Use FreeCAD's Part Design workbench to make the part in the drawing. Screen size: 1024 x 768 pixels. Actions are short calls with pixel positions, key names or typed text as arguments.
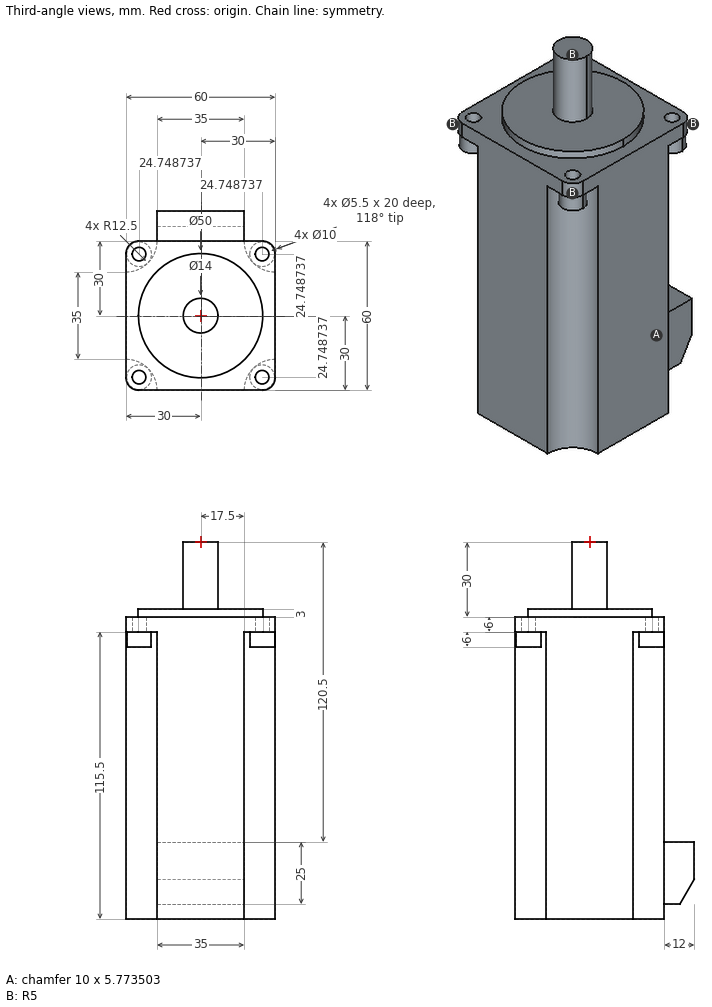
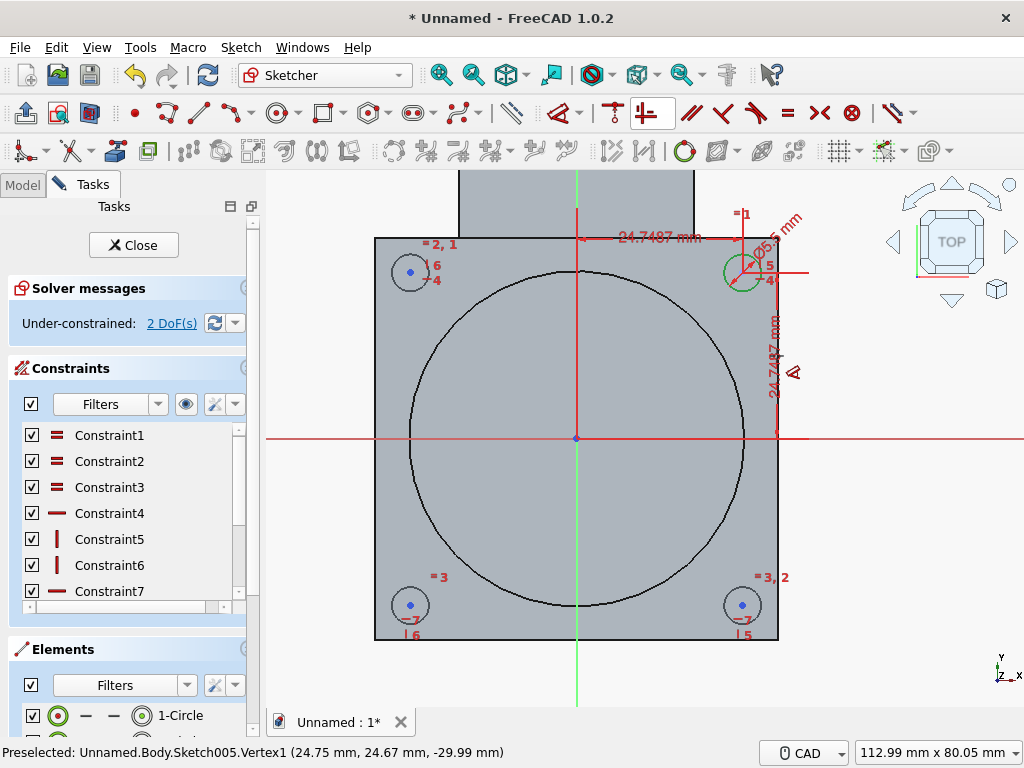
click(410, 273)
click(494, 239)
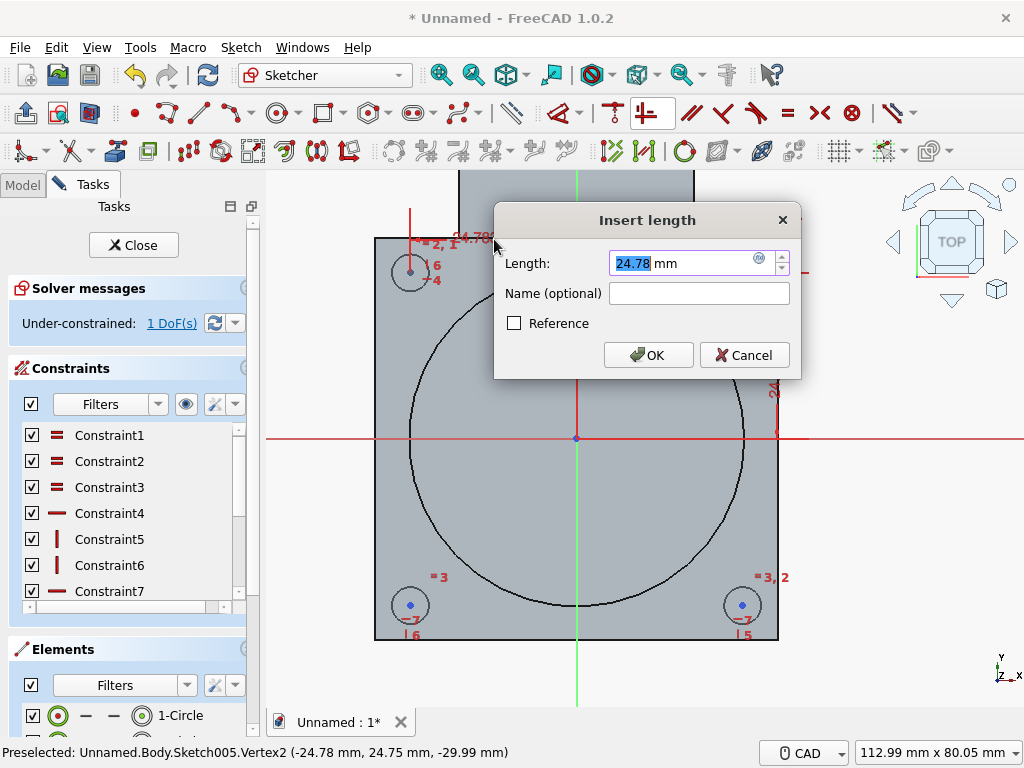
text(24.748737)
key(Return)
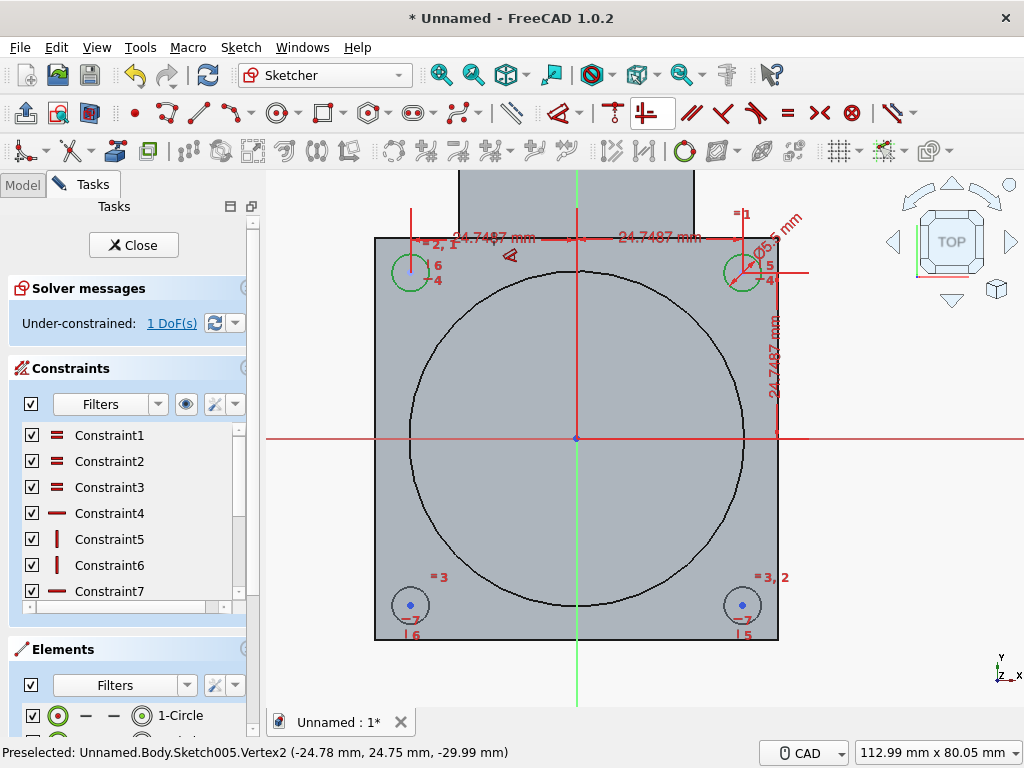
click(743, 606)
click(777, 522)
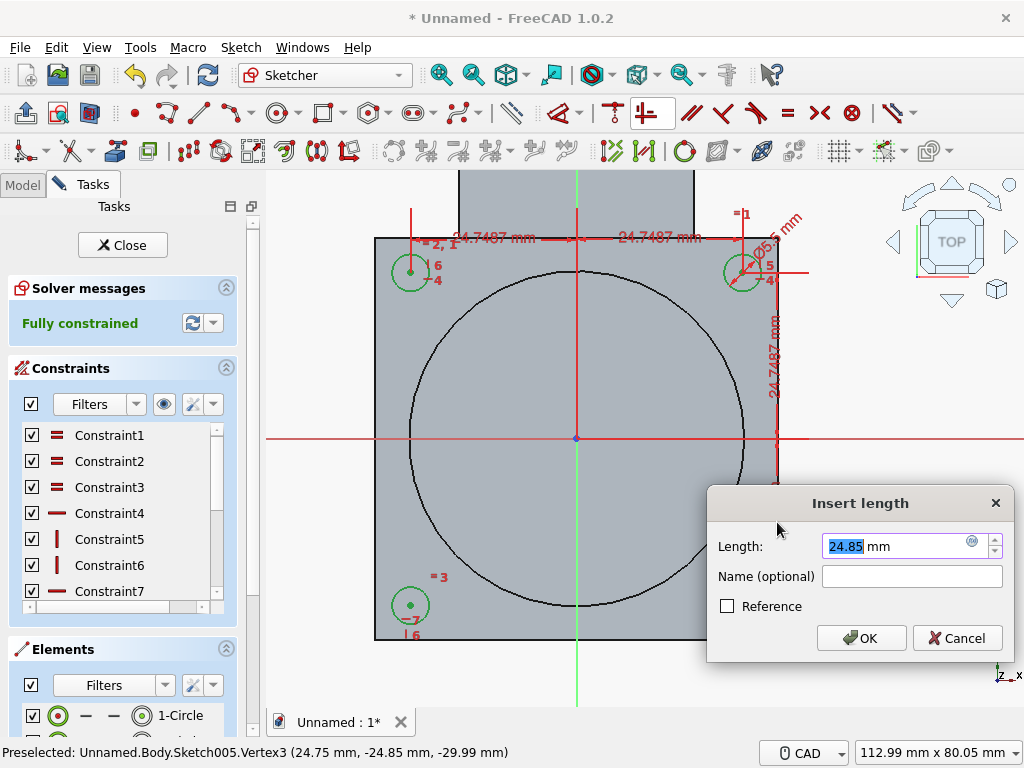
text(24.748737)
key(Return)
key(Escape)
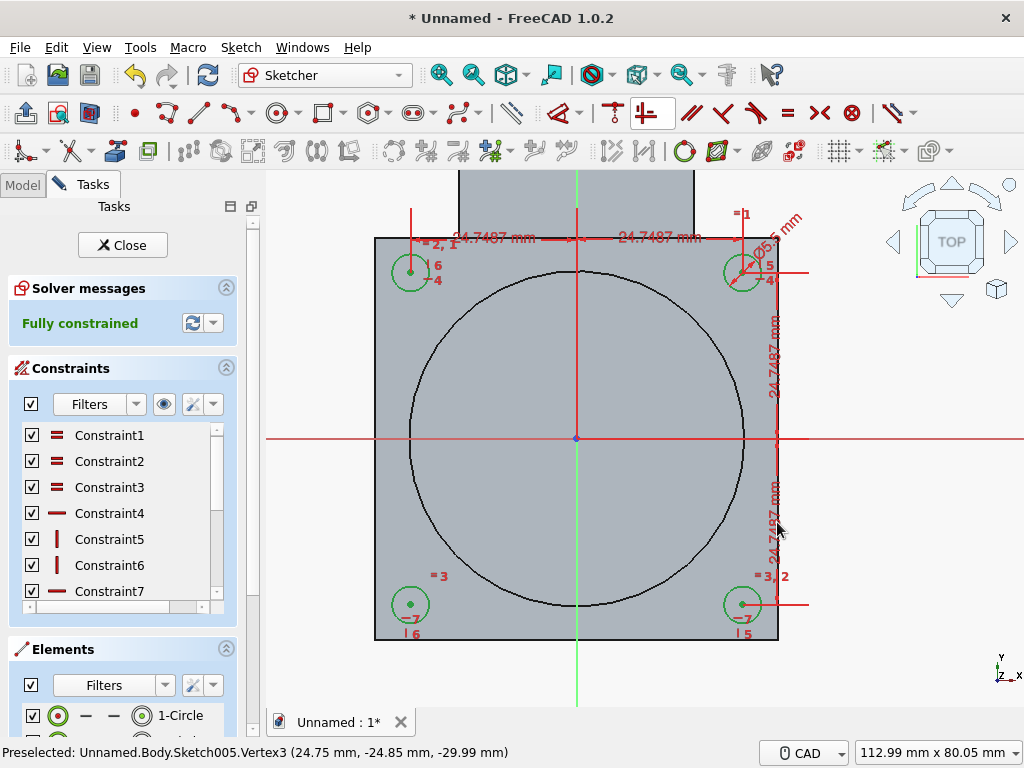
click(123, 245)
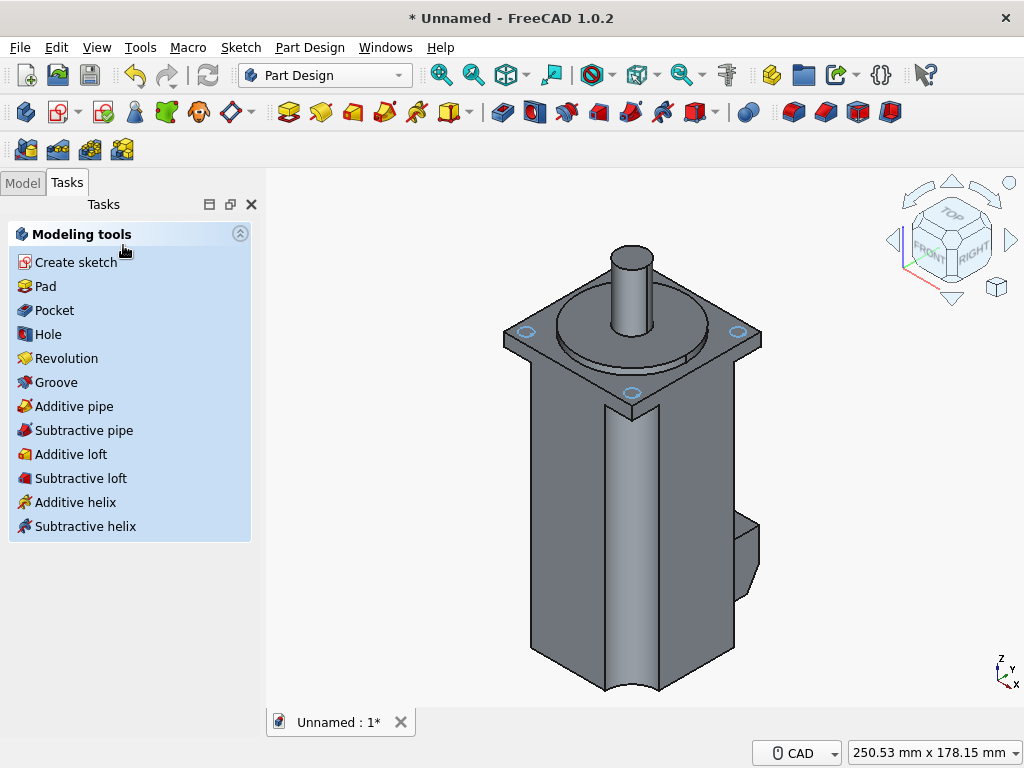
click(536, 112)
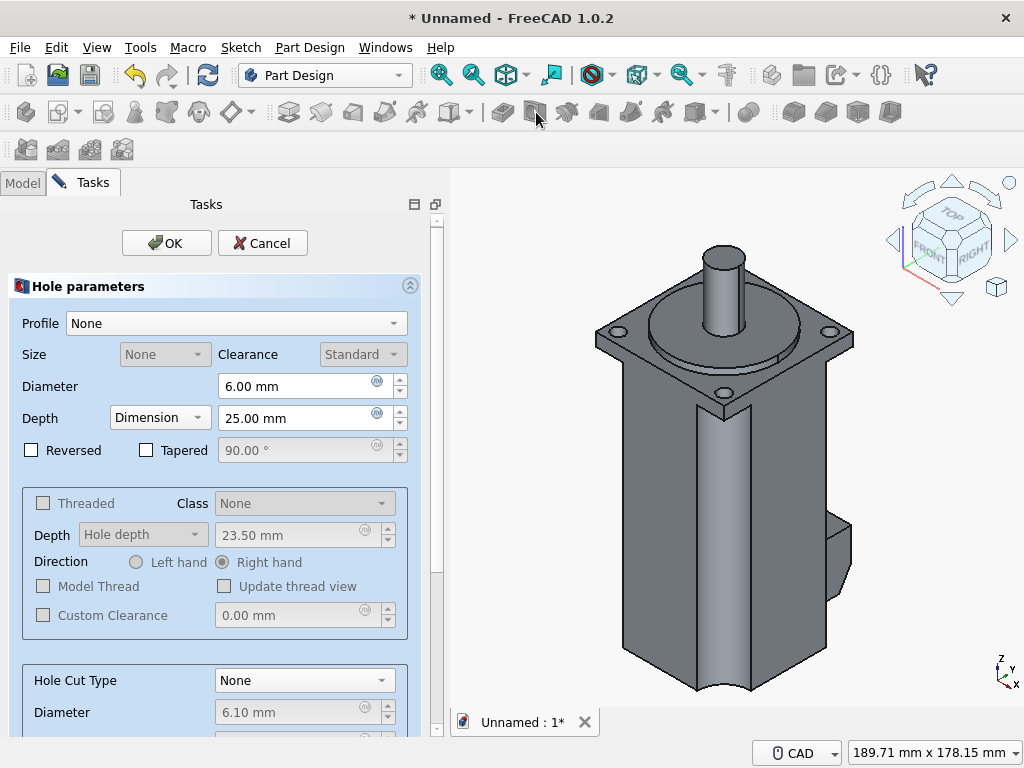
triple_click(305, 386)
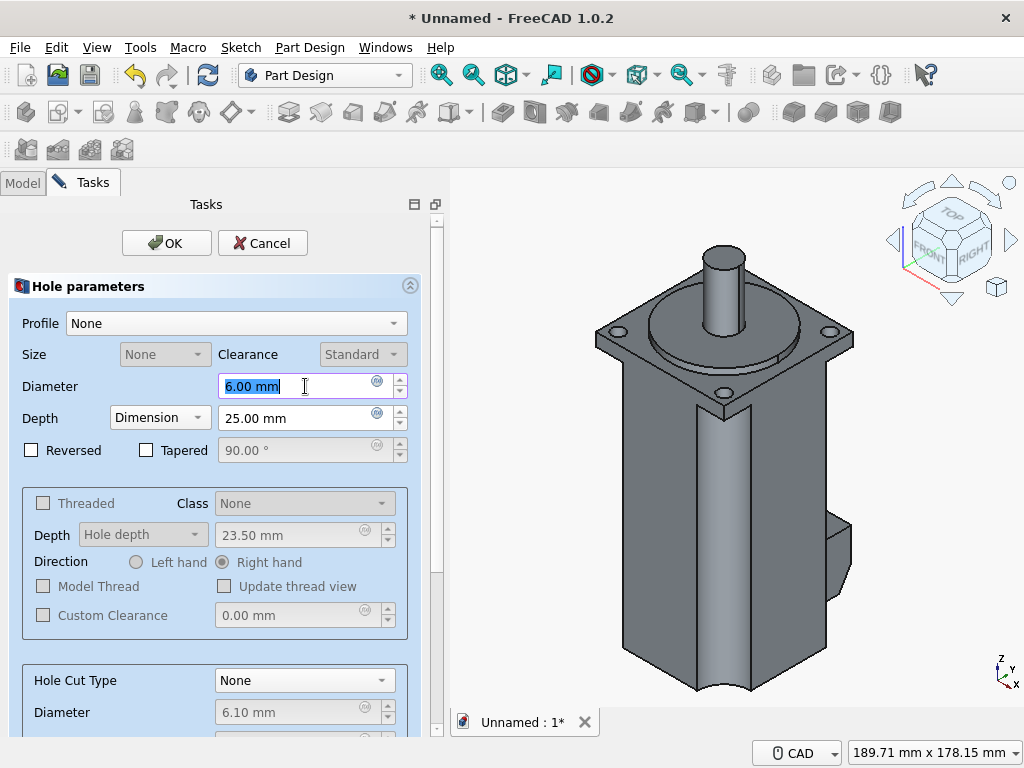
text(5.5)
key(Tab)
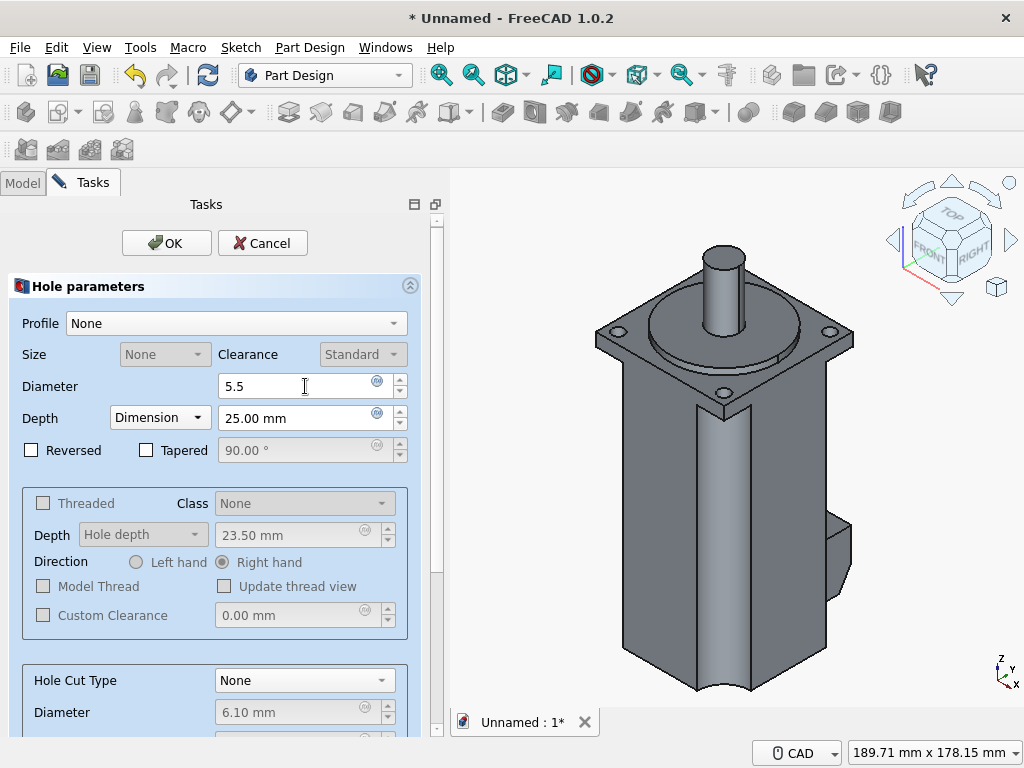
triple_click(305, 418)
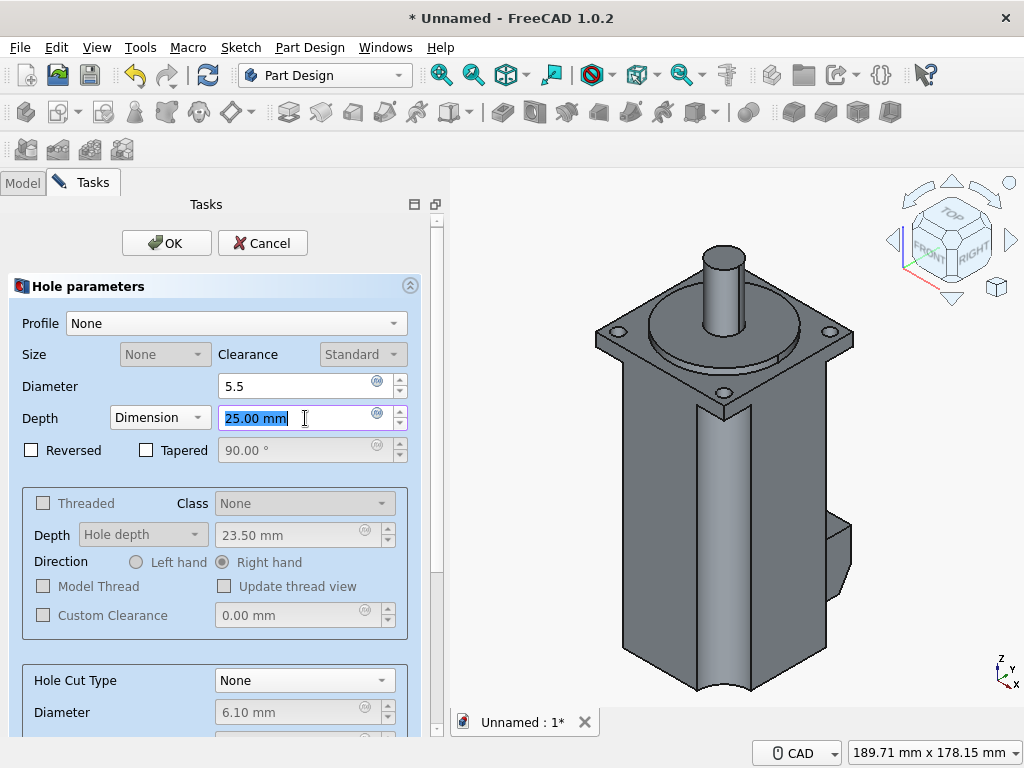
text(20)
key(Tab)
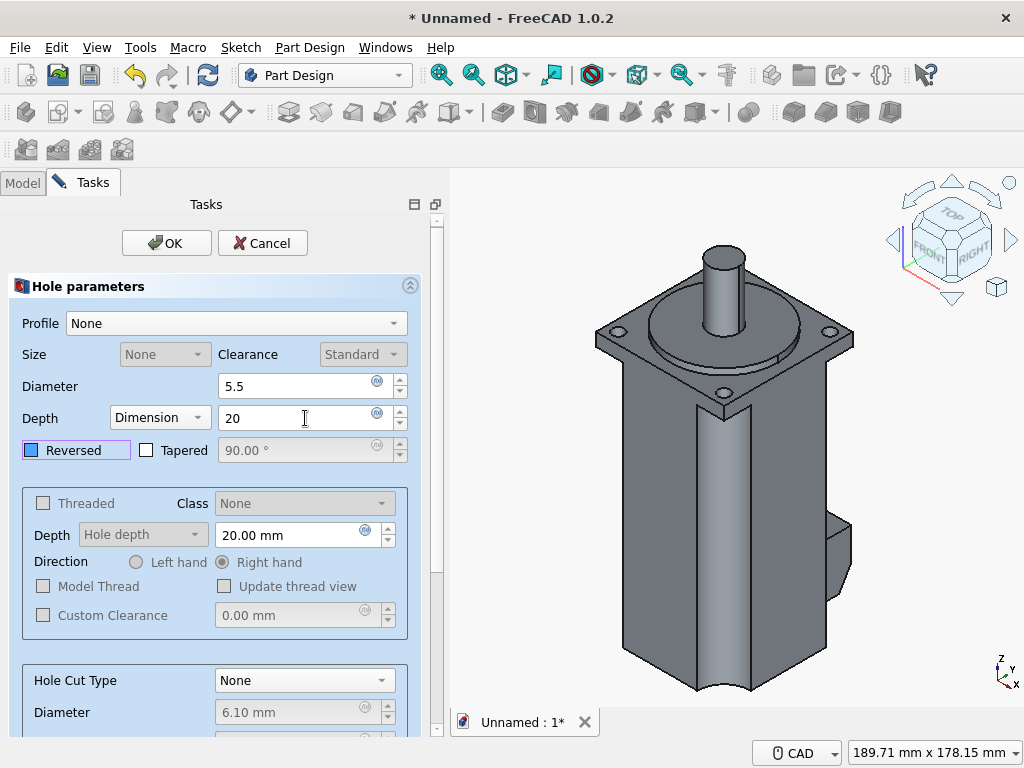
click(167, 243)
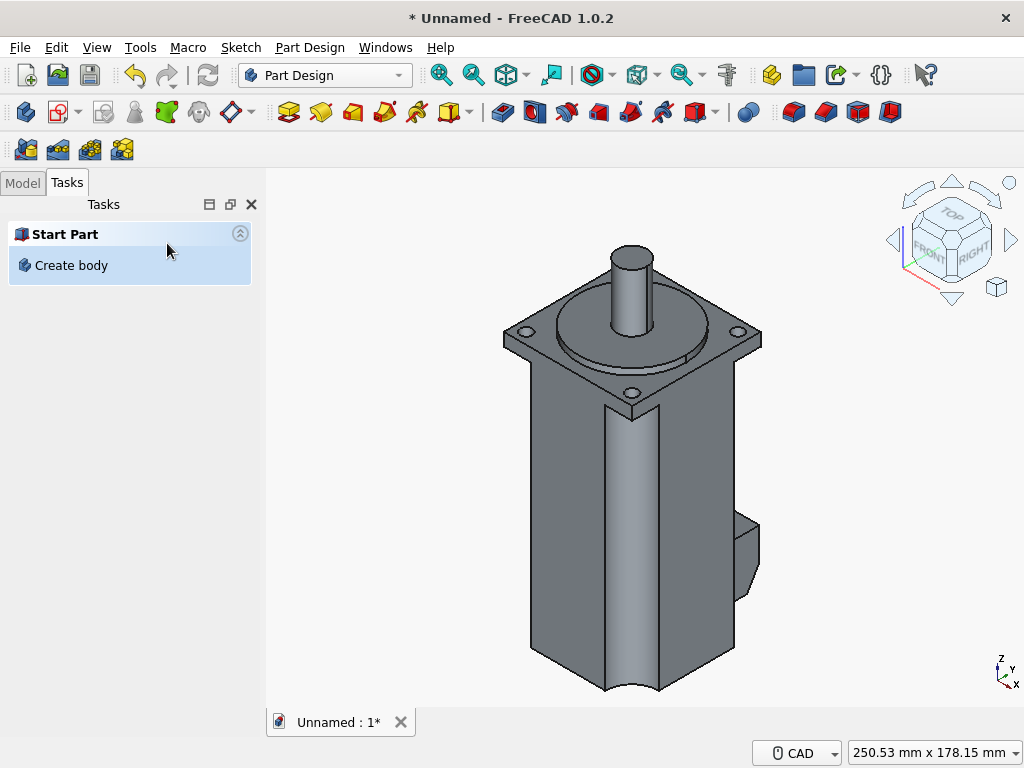
click(632, 412)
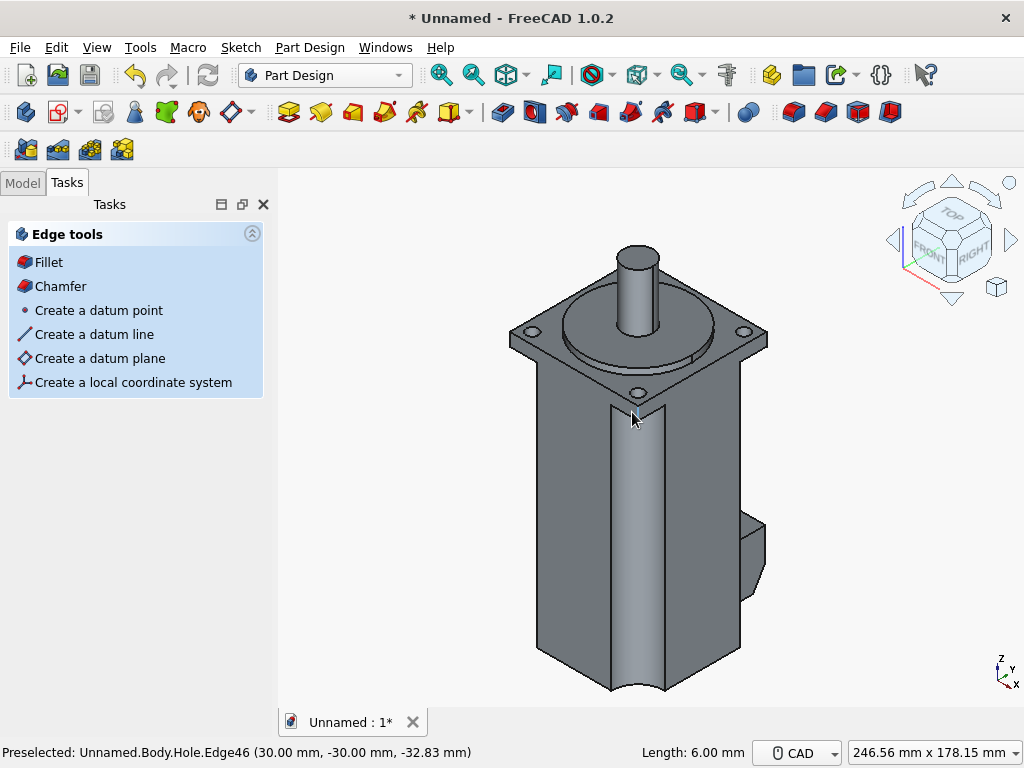
scroll(510, 338, up, 4)